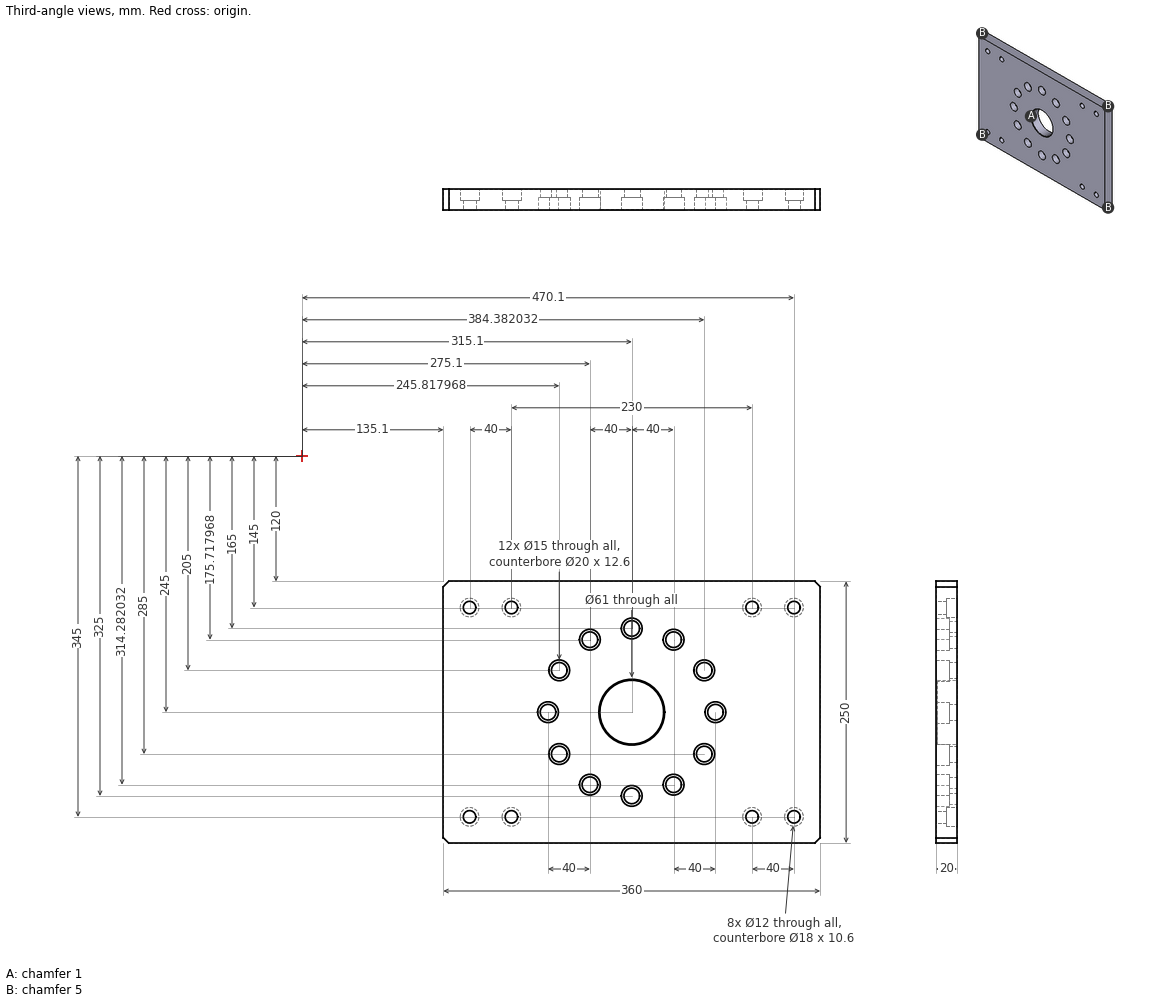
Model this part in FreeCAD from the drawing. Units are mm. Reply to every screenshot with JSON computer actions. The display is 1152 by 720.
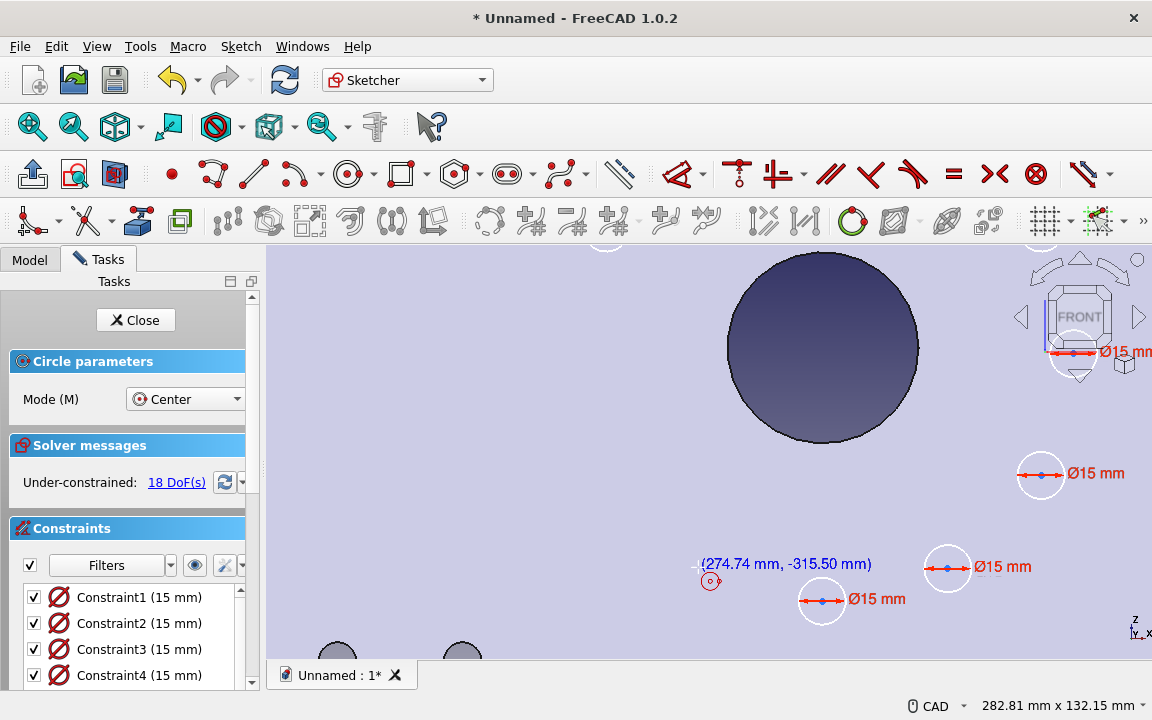
{"action": "scroll", "coordinate": [697, 567], "scroll_direction": "down", "scroll_amount": 7}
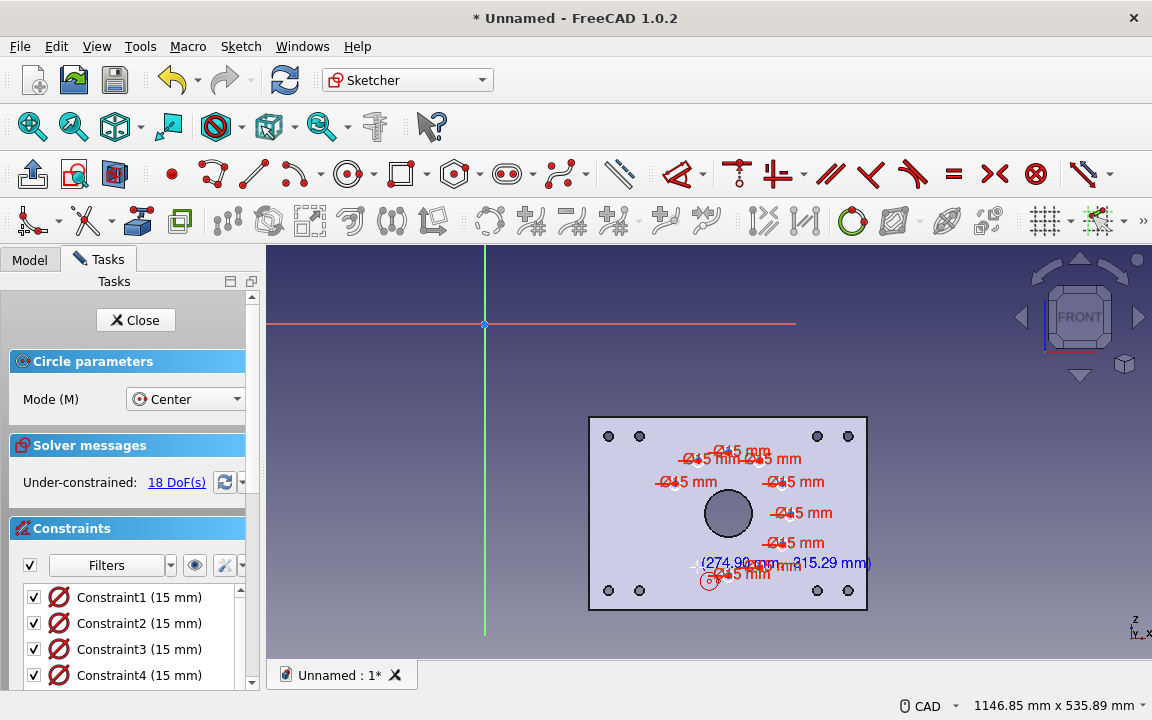
{"action": "left_click", "coordinate": [698, 567]}
{"action": "mouse_move", "coordinate": [702, 563]}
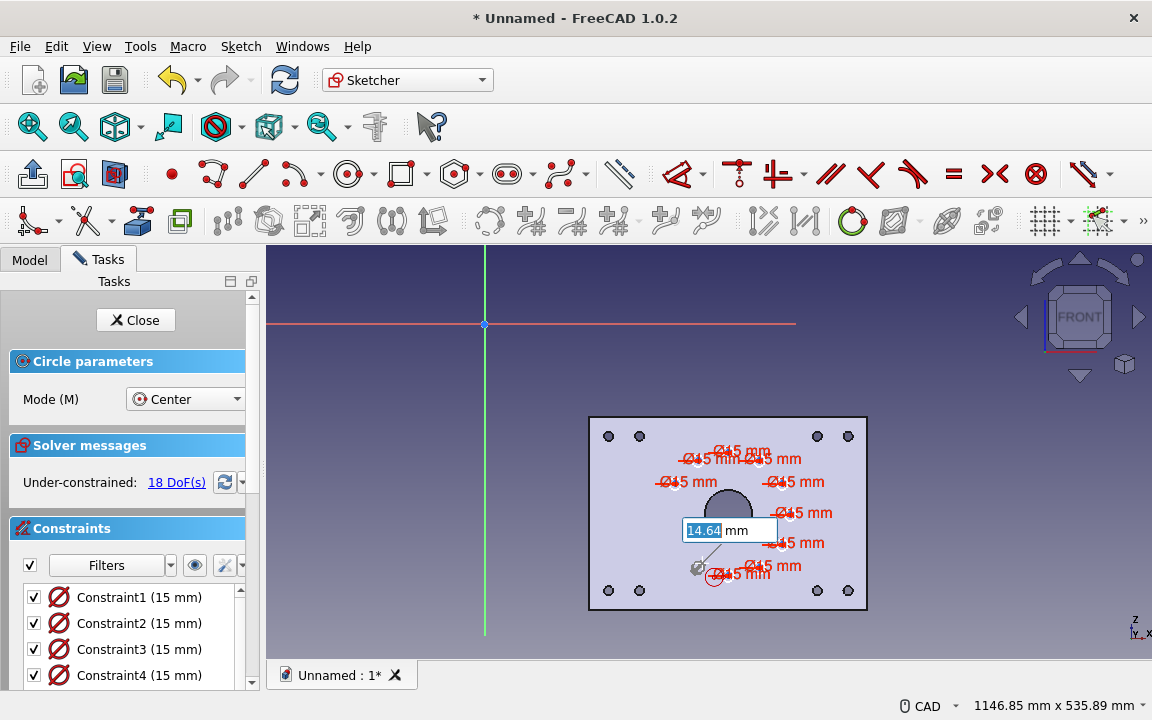
{"action": "type", "text": "15"}
{"action": "key", "text": "Return"}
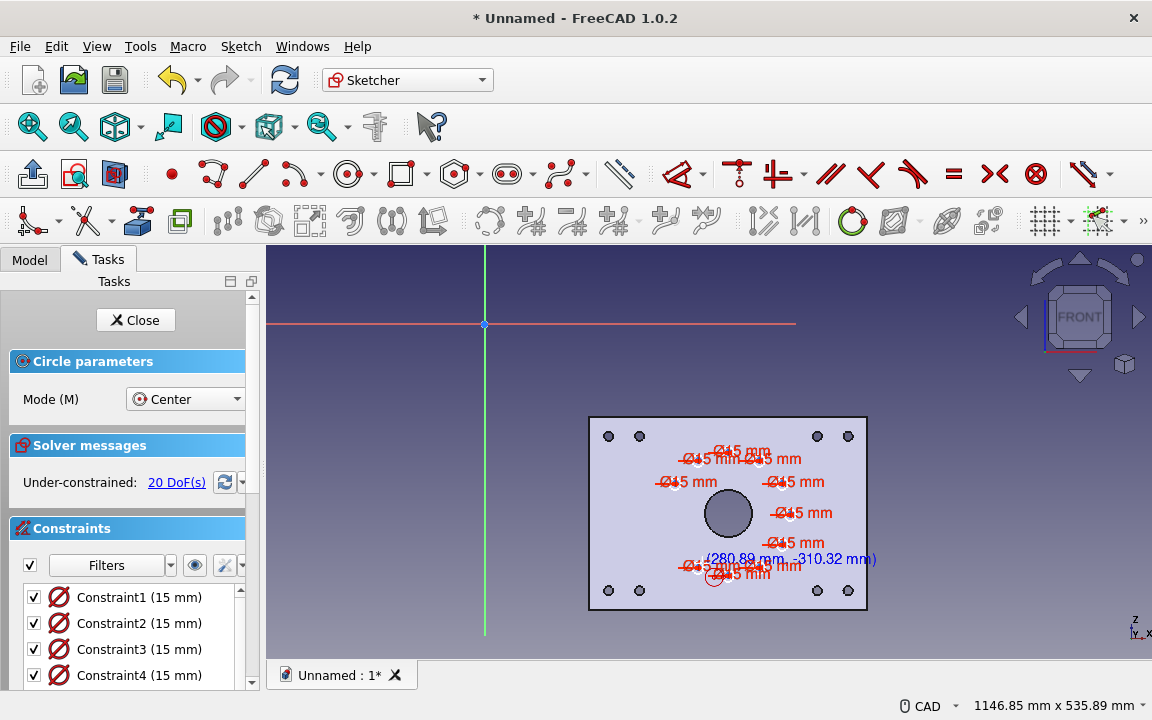
{"action": "scroll", "coordinate": [675, 544], "scroll_direction": "up", "scroll_amount": 7}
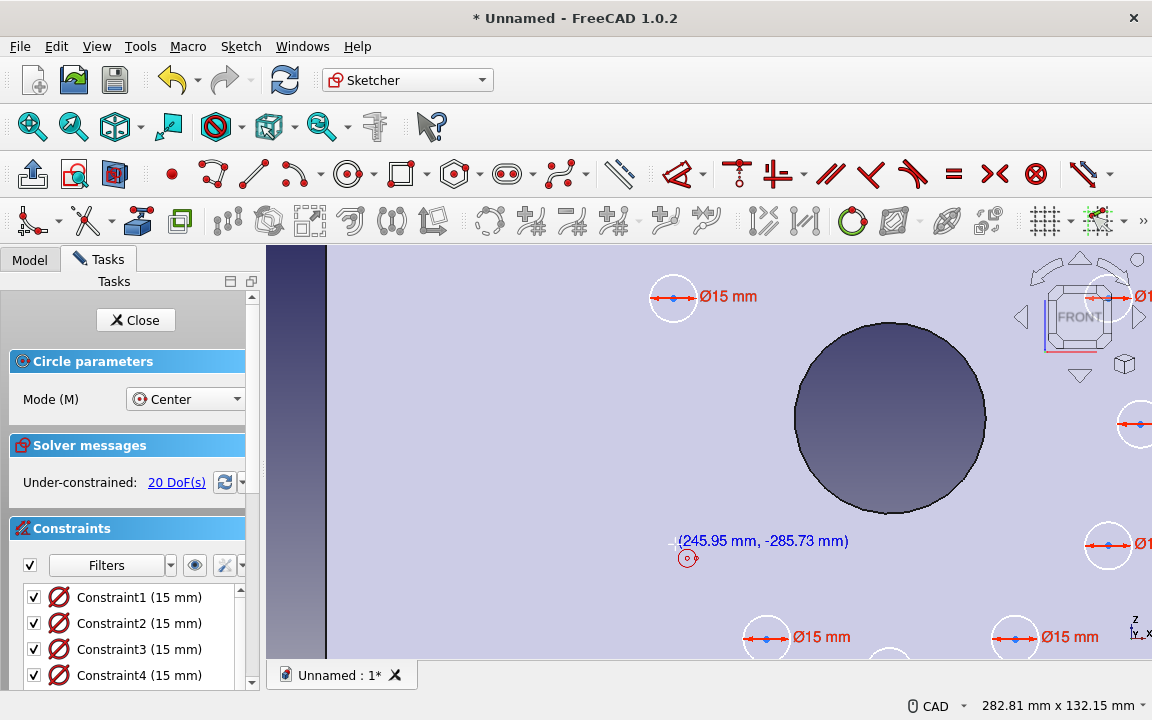
{"action": "scroll", "coordinate": [675, 544], "scroll_direction": "down", "scroll_amount": 7}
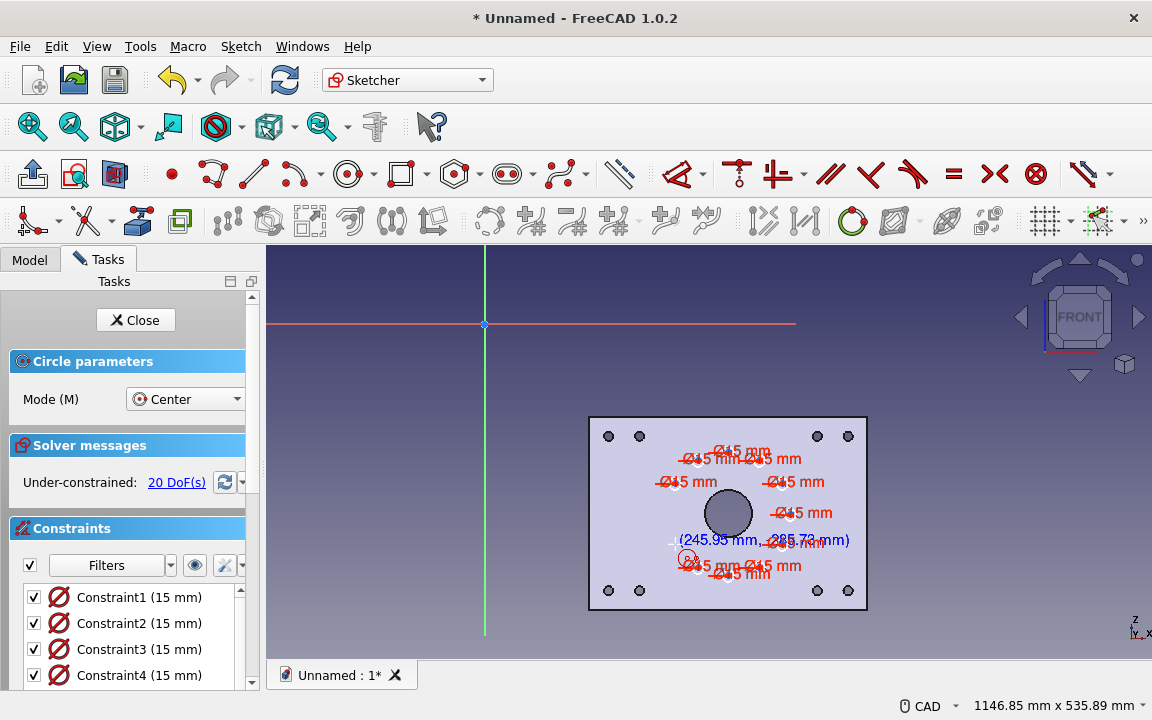
{"action": "left_click", "coordinate": [675, 544]}
{"action": "mouse_move", "coordinate": [679, 540]}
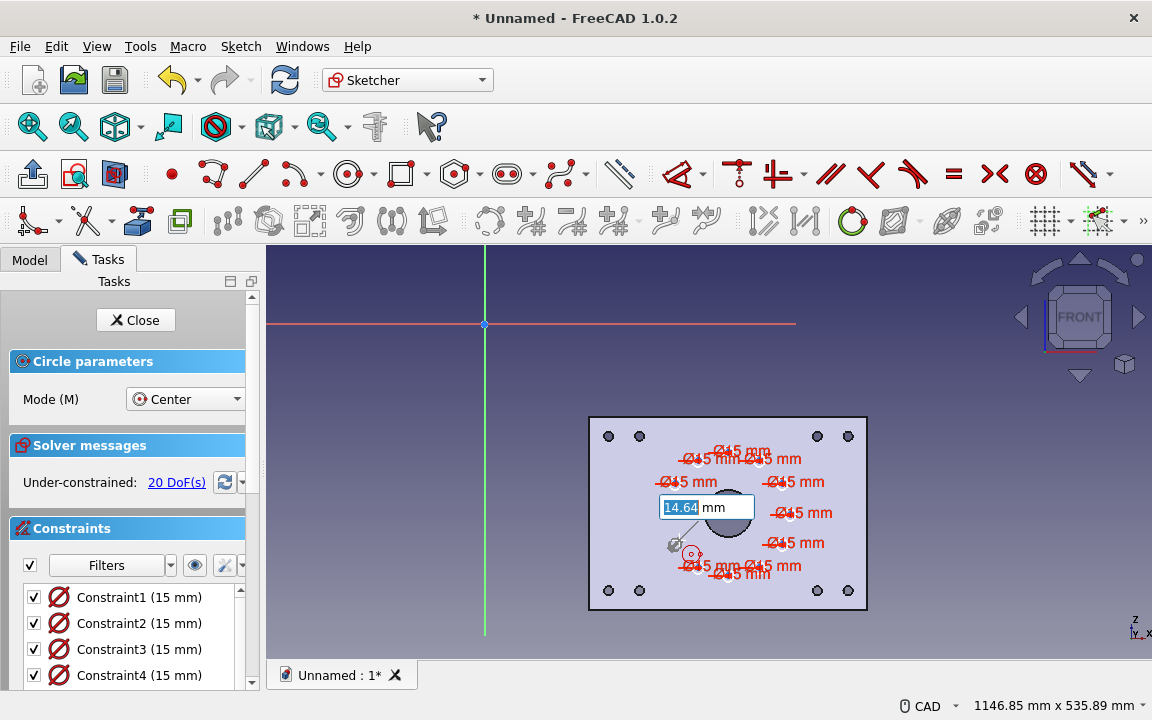
{"action": "type", "text": "15"}
{"action": "key", "text": "Return"}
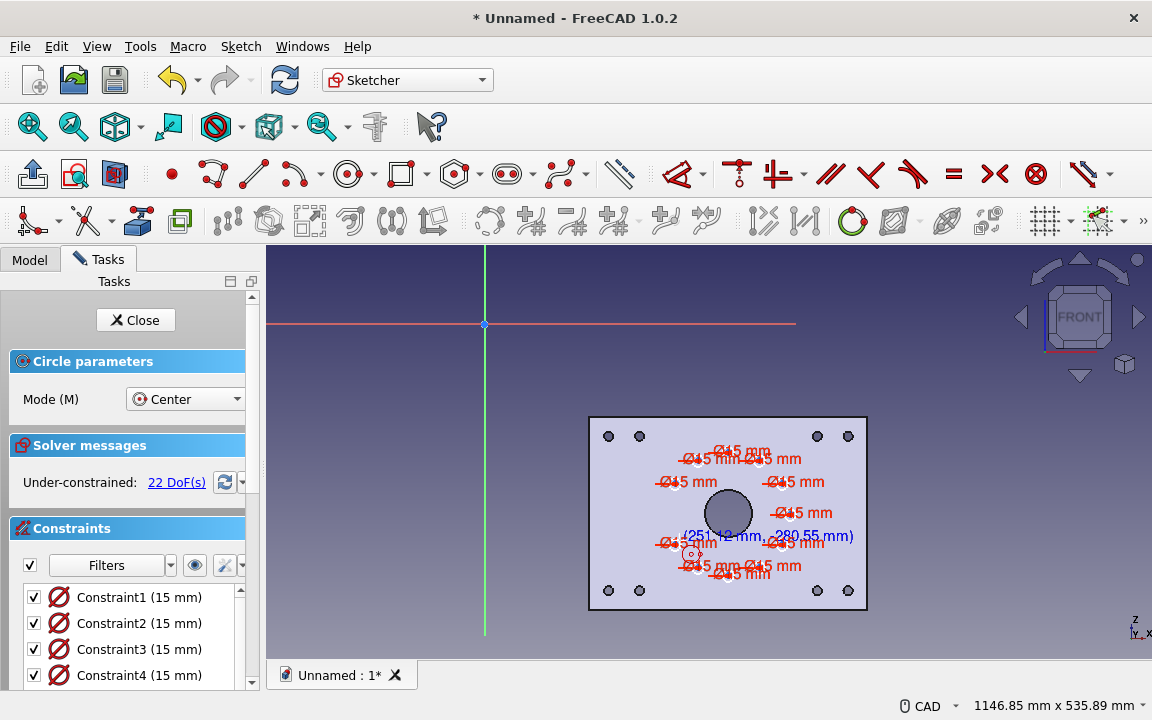
{"action": "scroll", "coordinate": [667, 514], "scroll_direction": "up", "scroll_amount": 7}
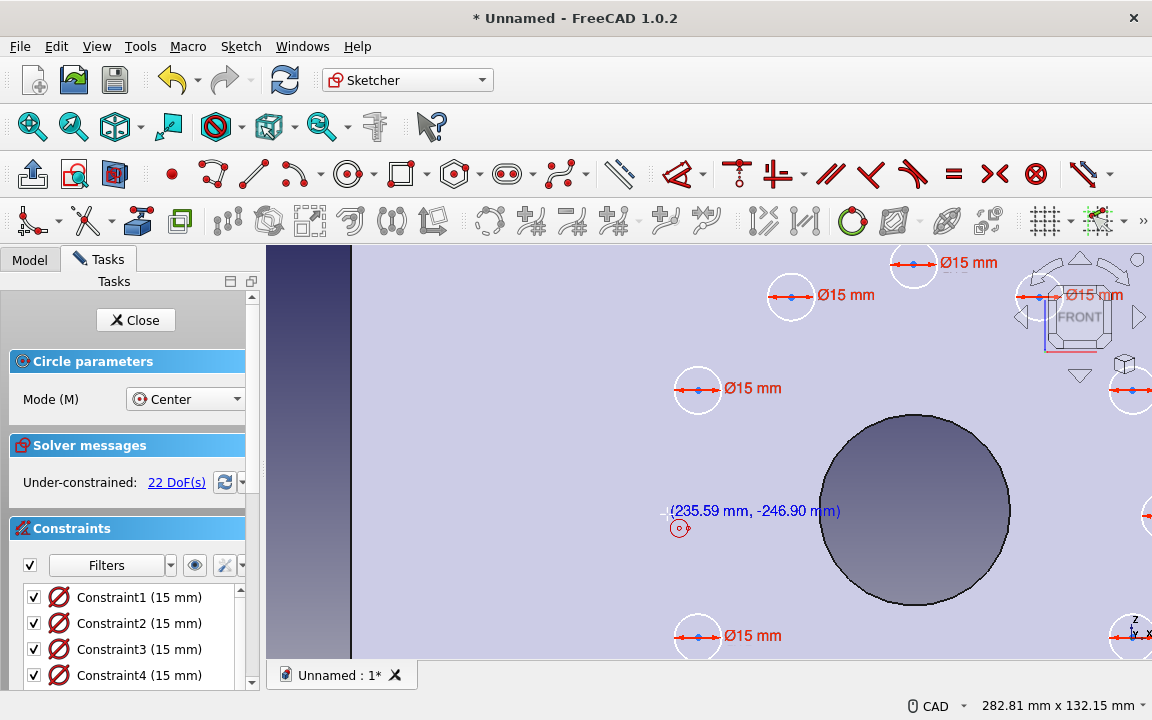
{"action": "scroll", "coordinate": [667, 514], "scroll_direction": "down", "scroll_amount": 7}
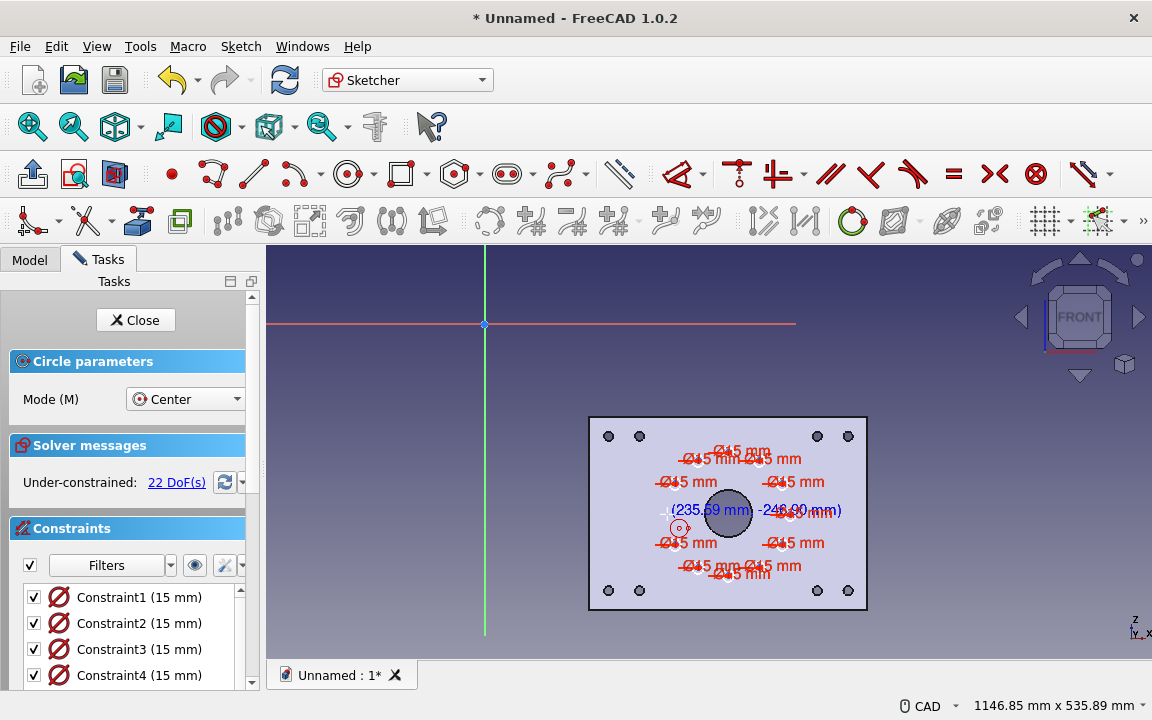
{"action": "left_click", "coordinate": [667, 514]}
{"action": "mouse_move", "coordinate": [671, 509]}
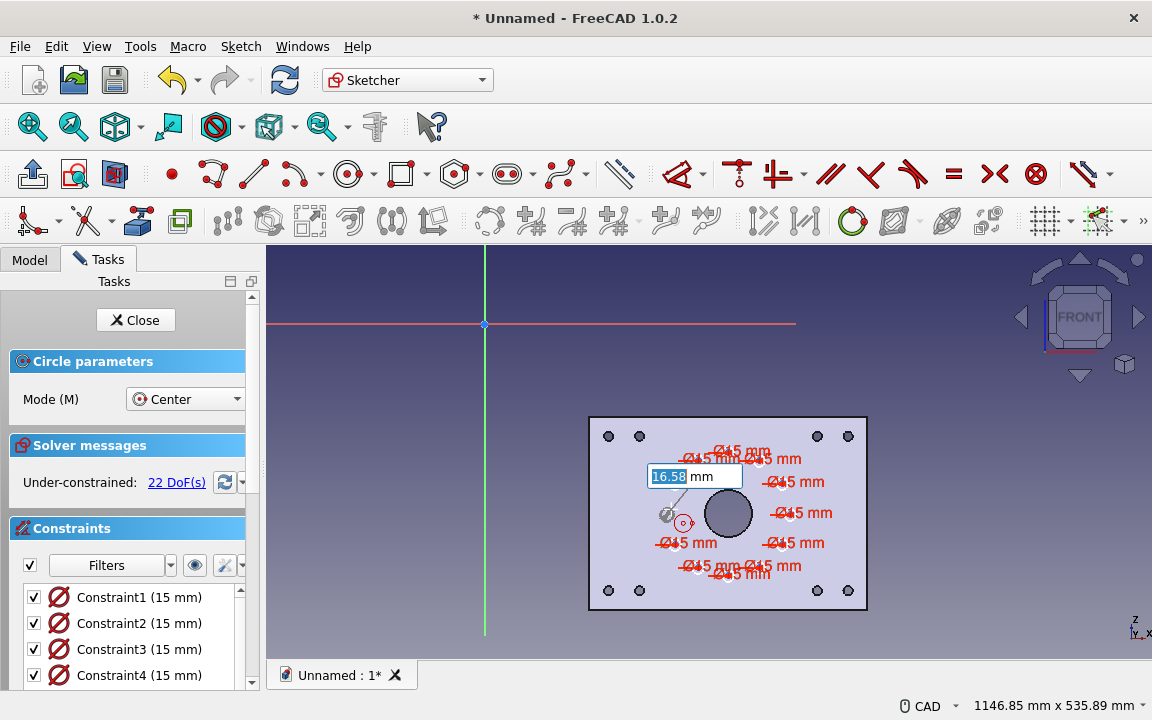
{"action": "type", "text": "15"}
{"action": "key", "text": "Return"}
{"action": "key", "text": "Escape"}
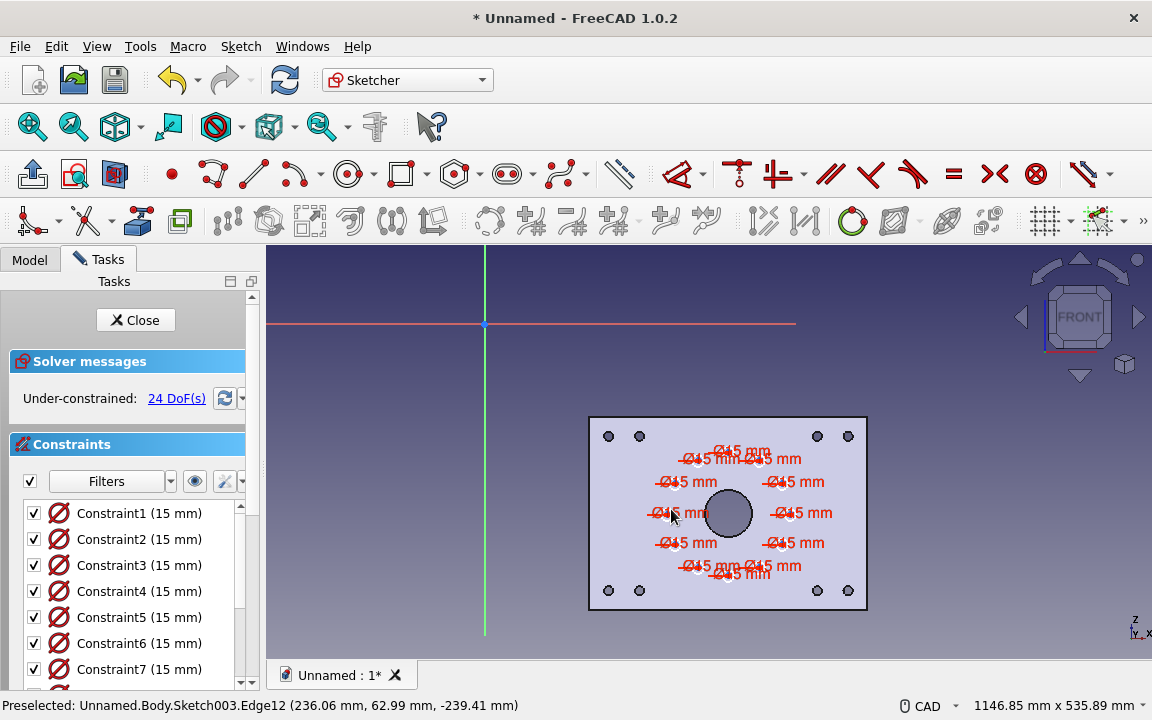
{"action": "left_click", "coordinate": [676, 174]}